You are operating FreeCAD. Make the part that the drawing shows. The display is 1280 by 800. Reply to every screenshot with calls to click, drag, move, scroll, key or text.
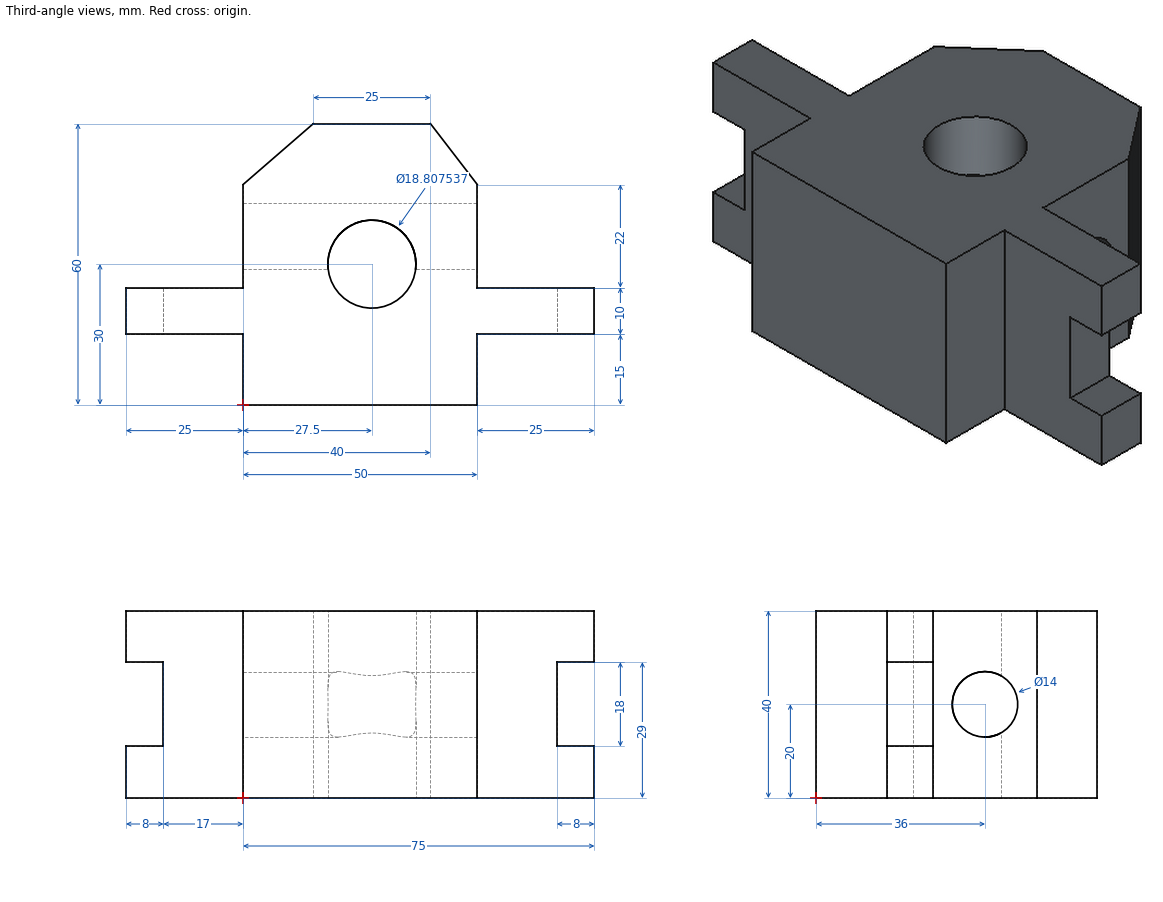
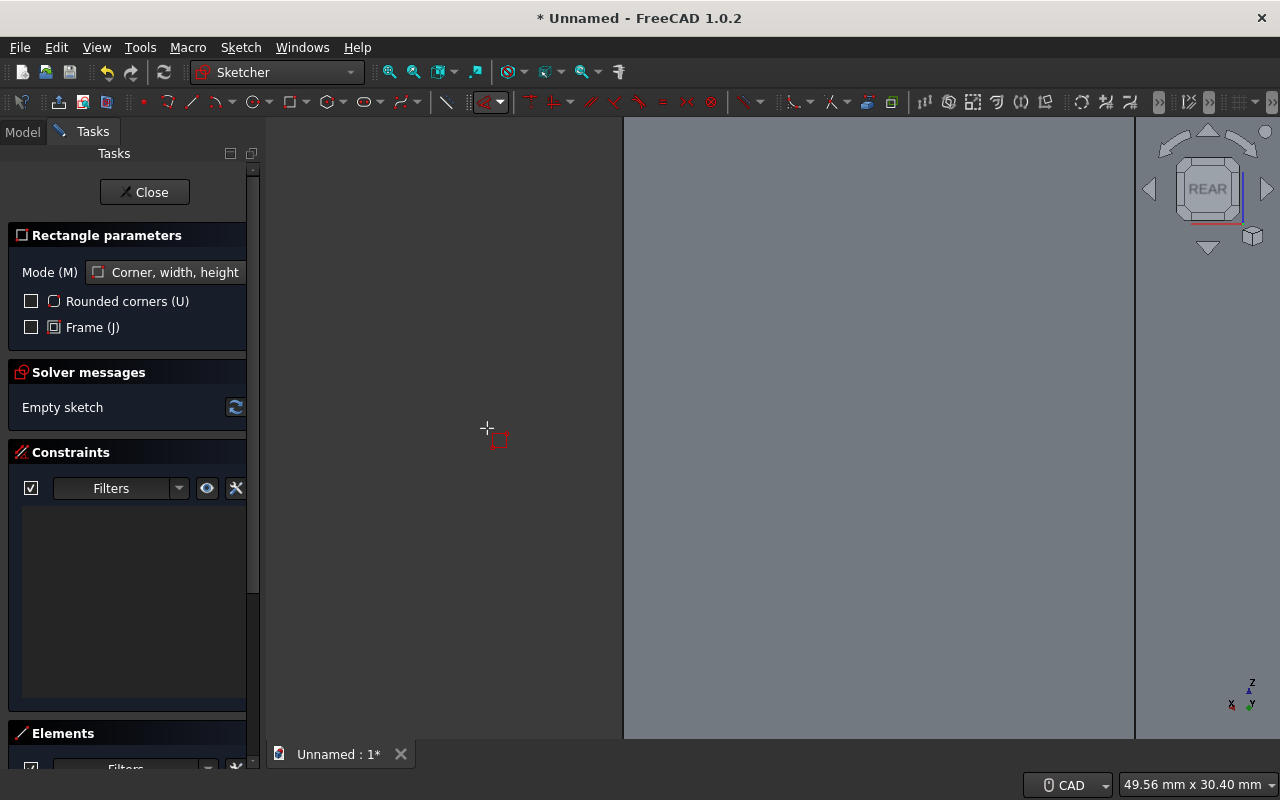
click(623, 242)
move(787, 611)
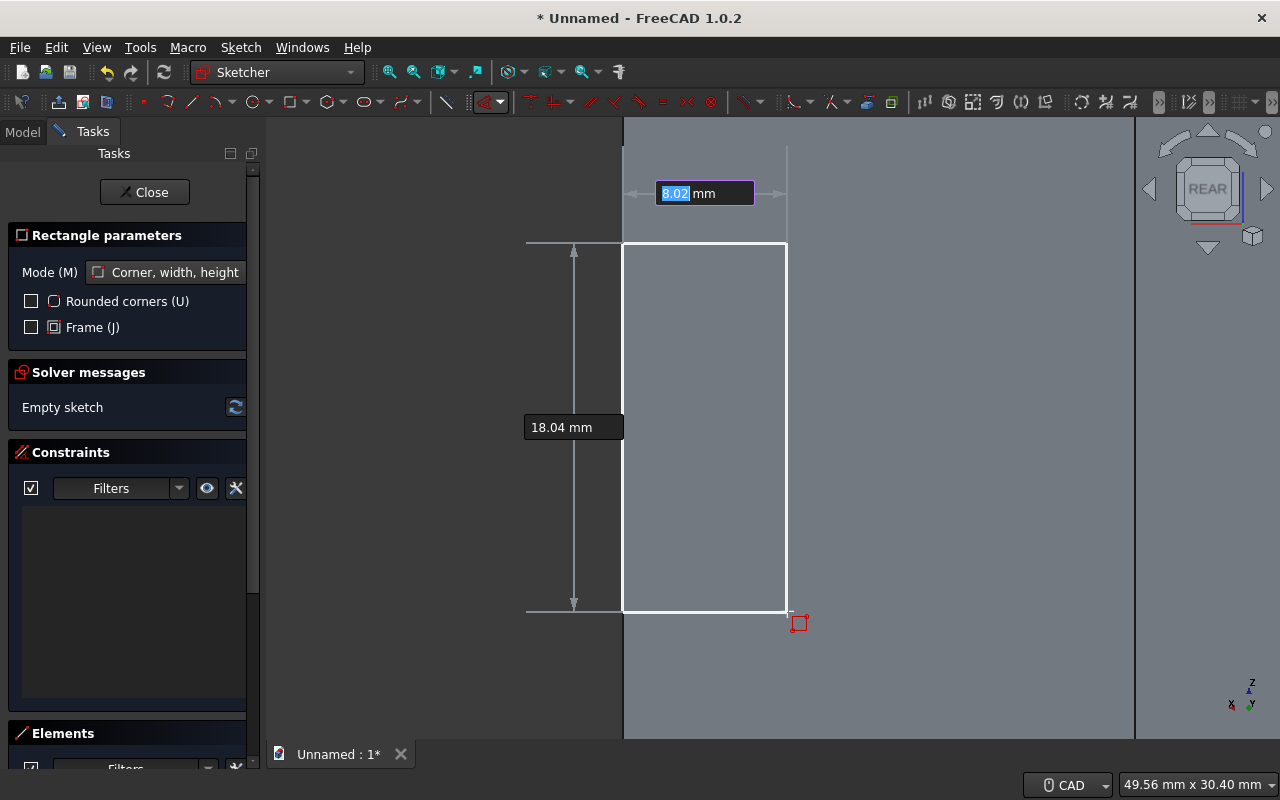
text(8)
key(Tab)
text(18)
key(Return)
key(Escape)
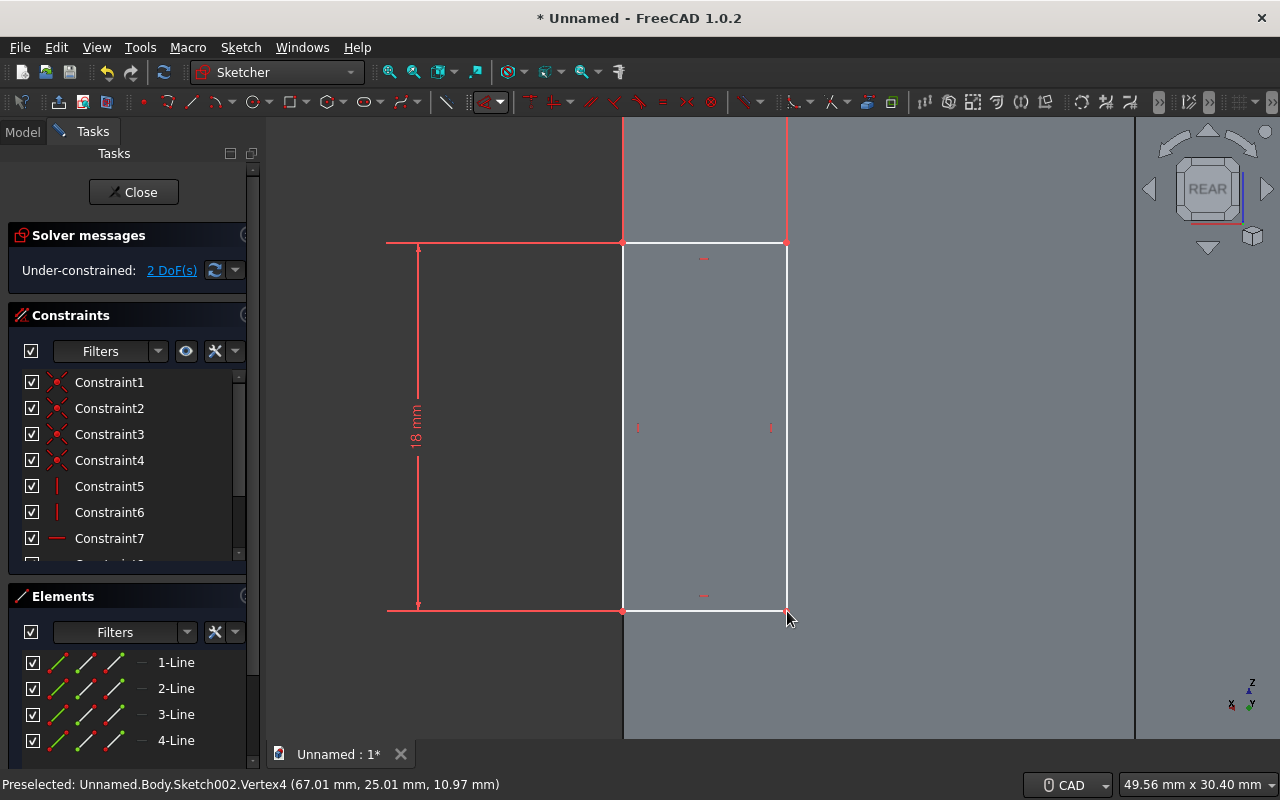
click(623, 243)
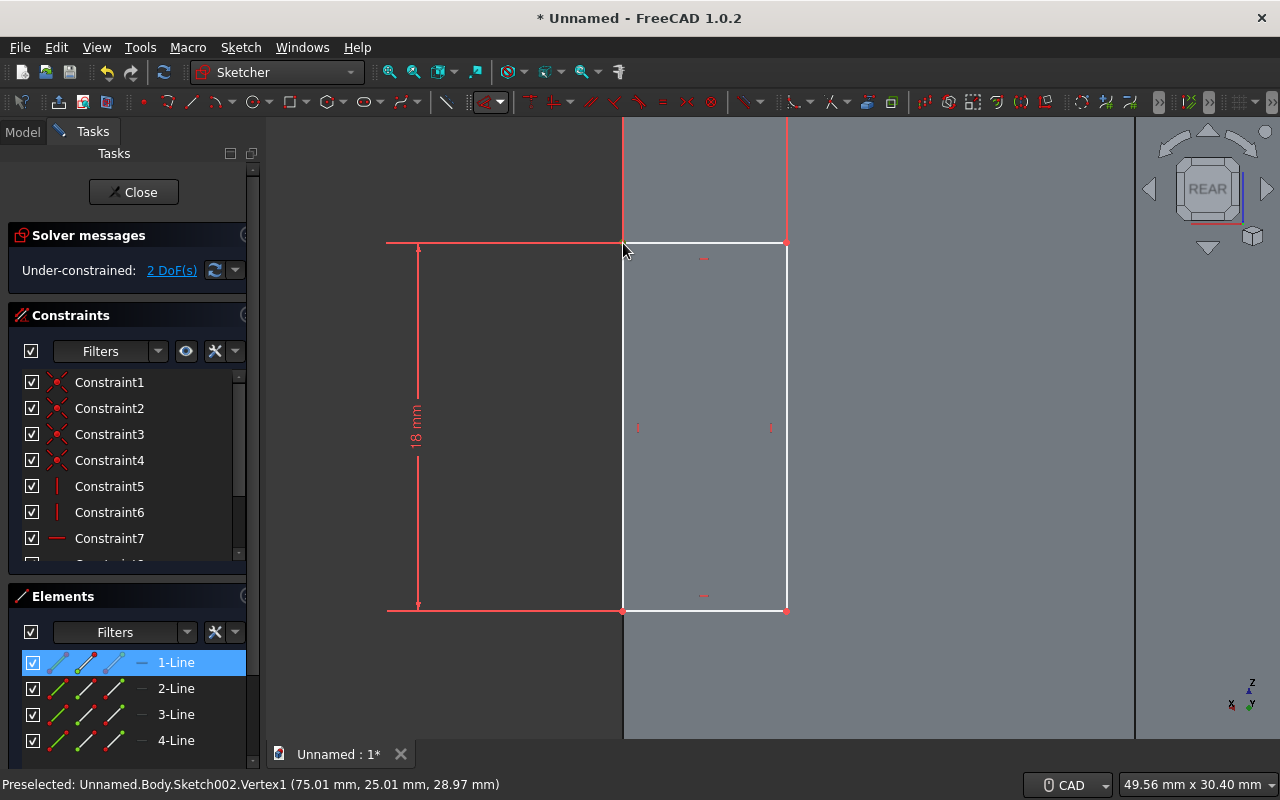
key(l)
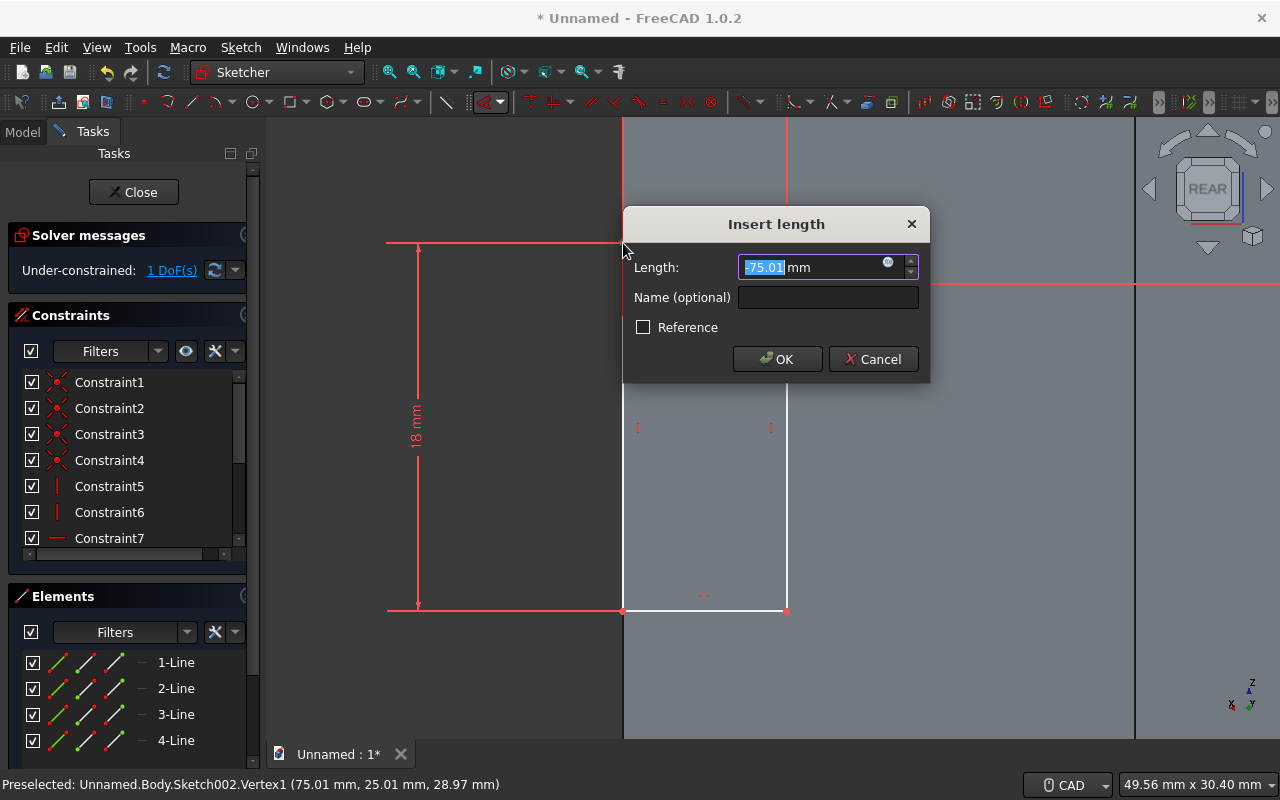
text(-75)
key(Return)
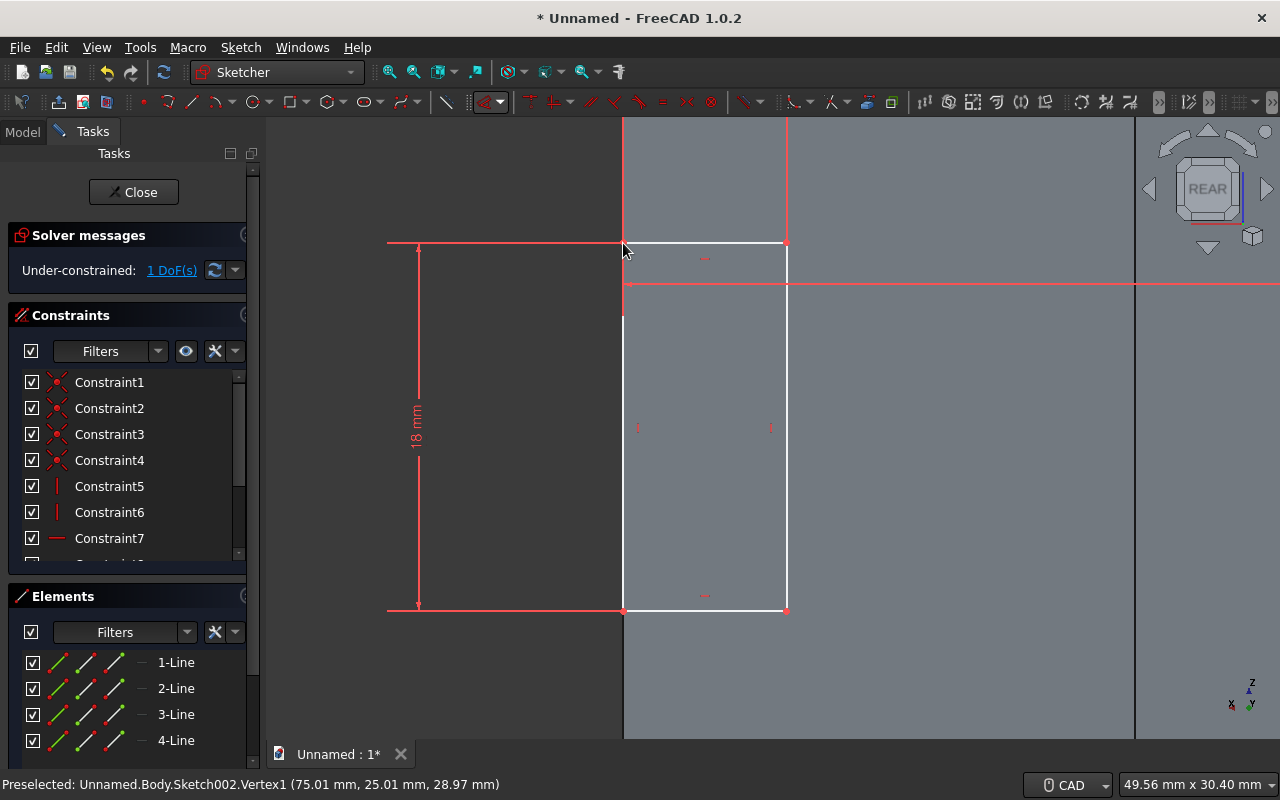
click(623, 243)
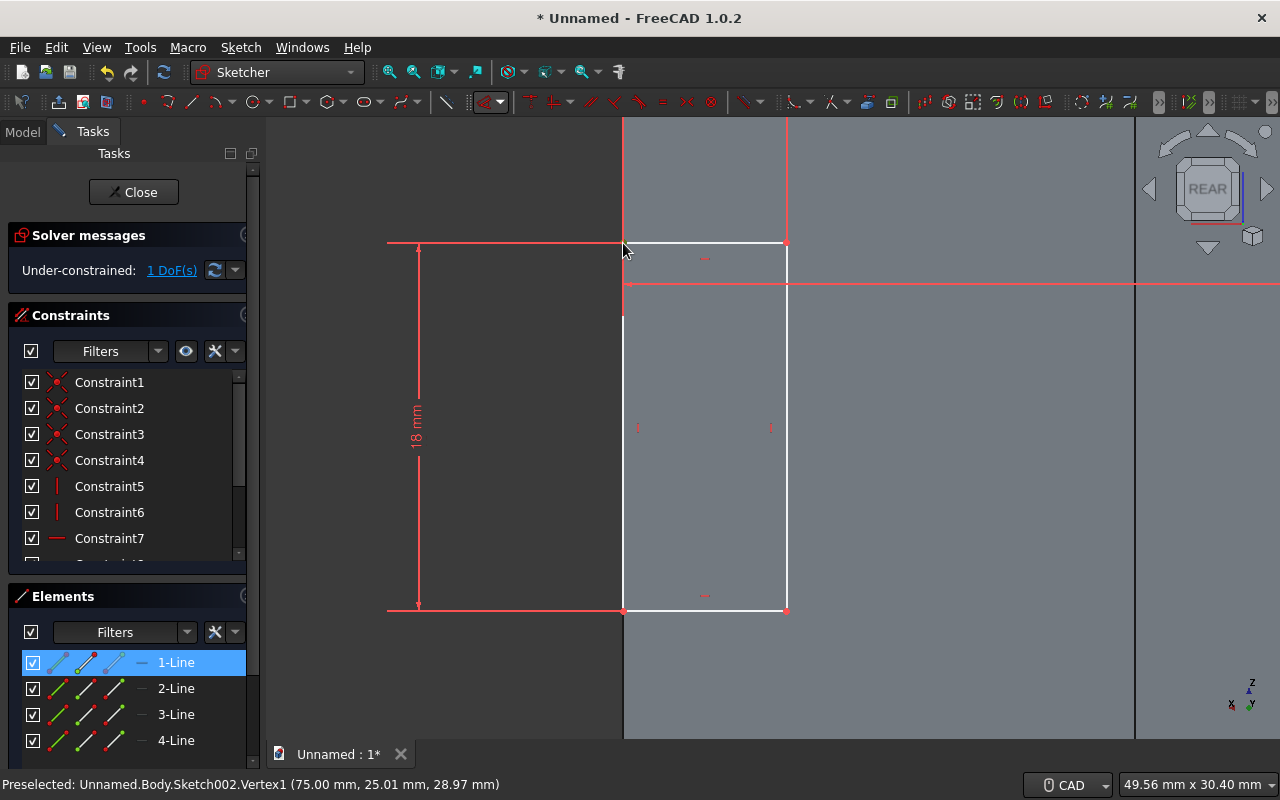
key(i)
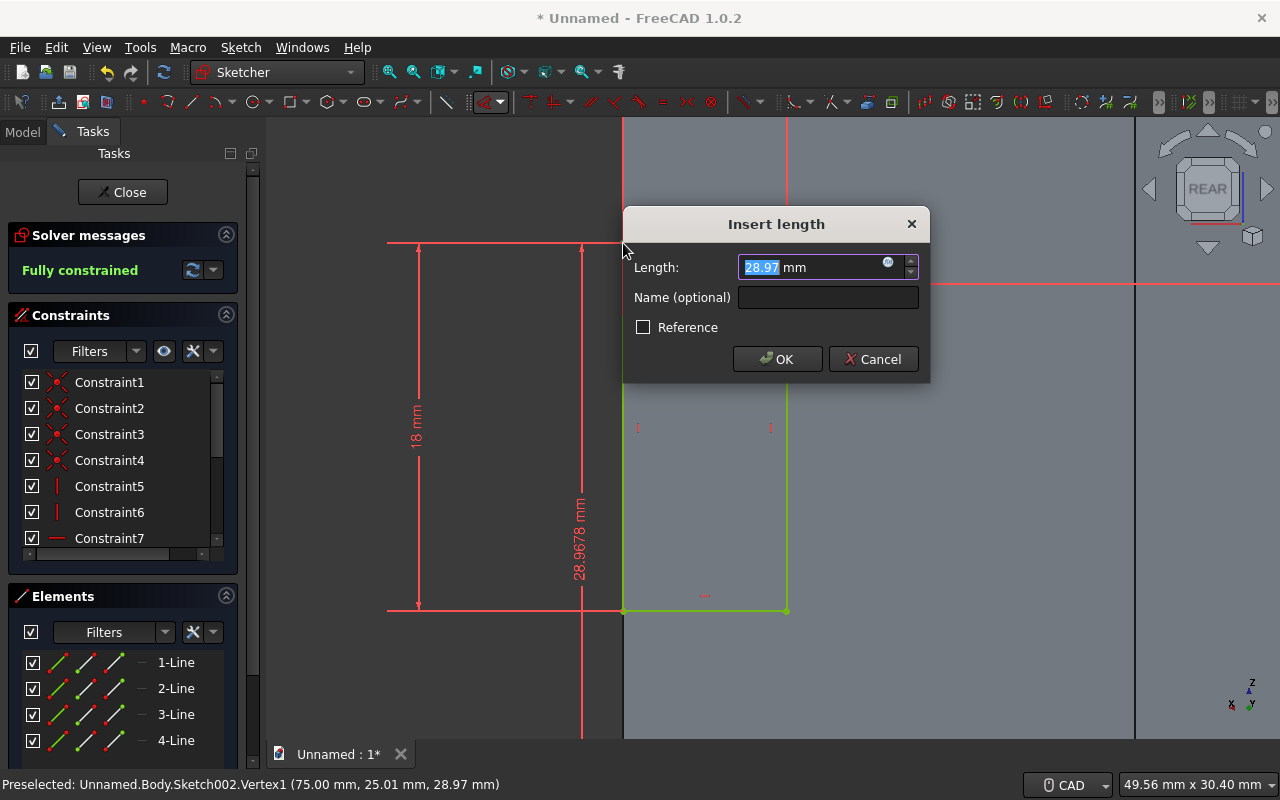
text(29)
key(Return)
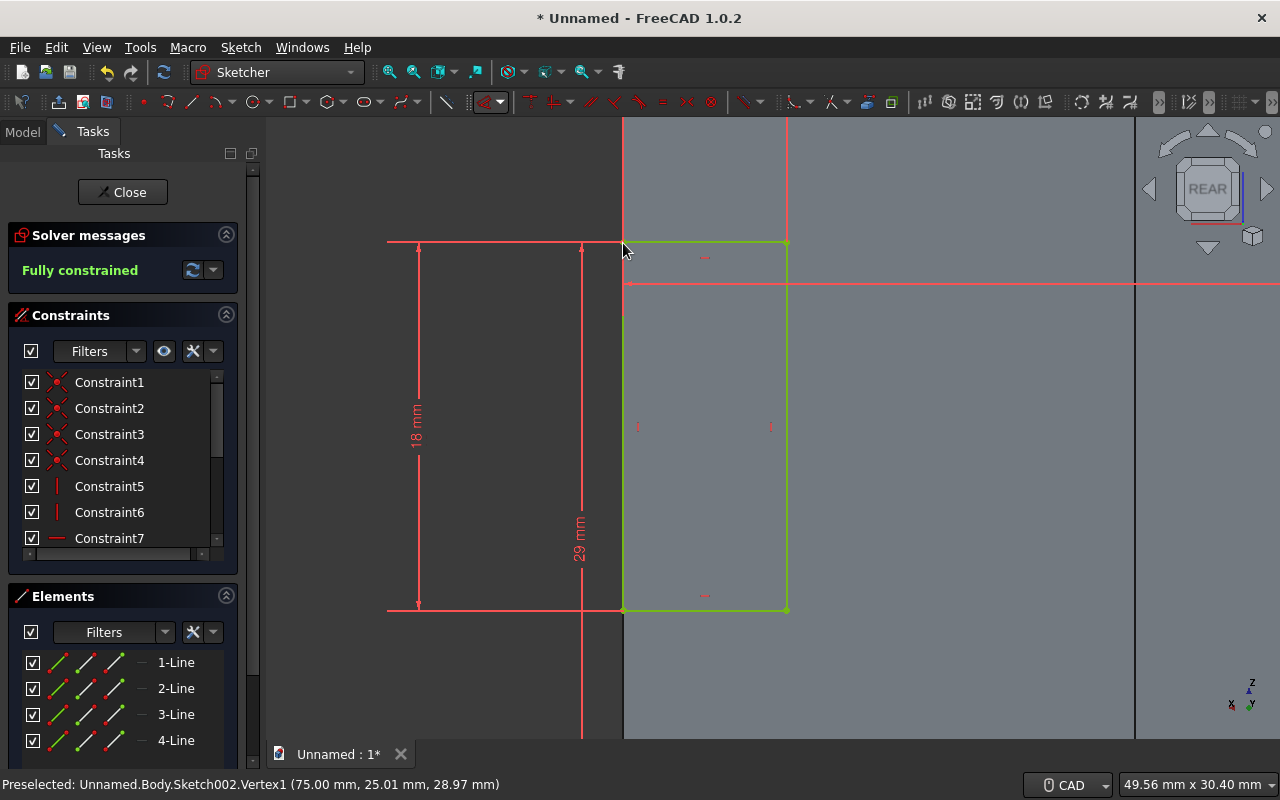
click(123, 192)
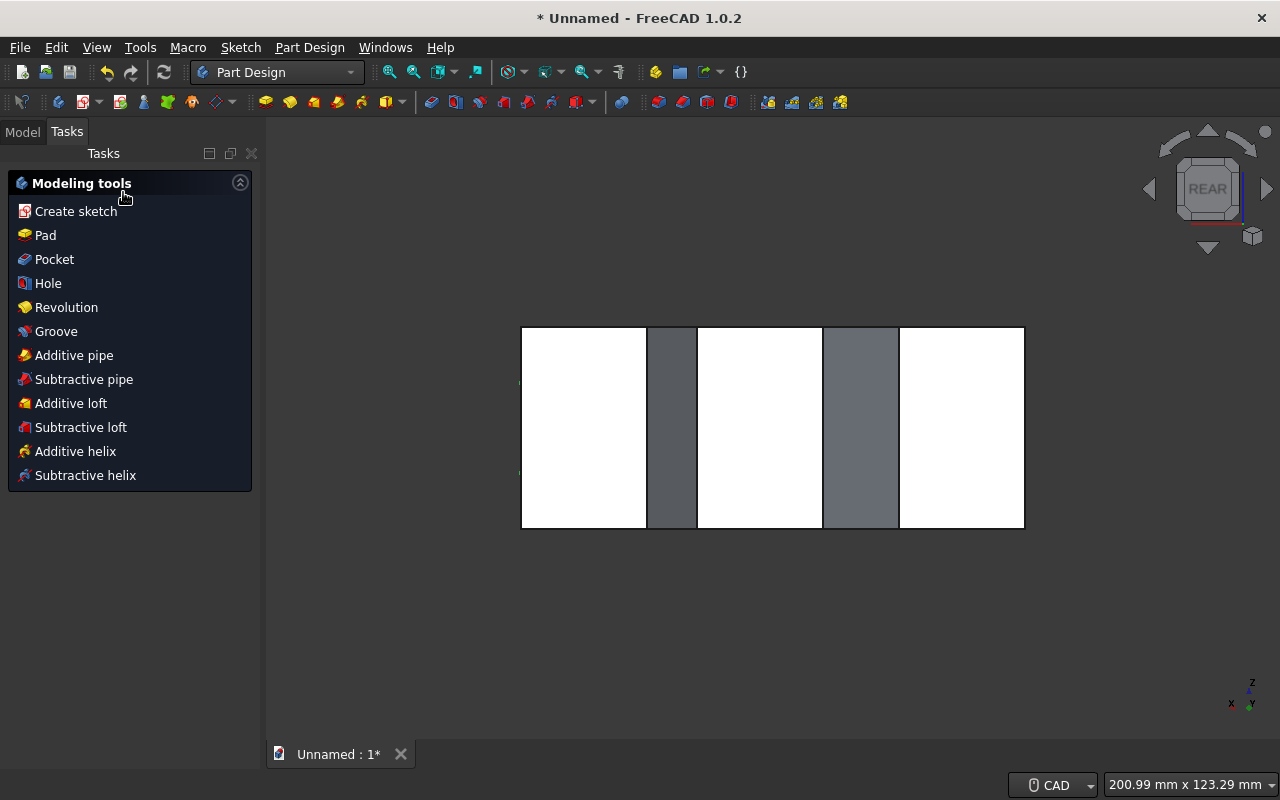
click(432, 102)